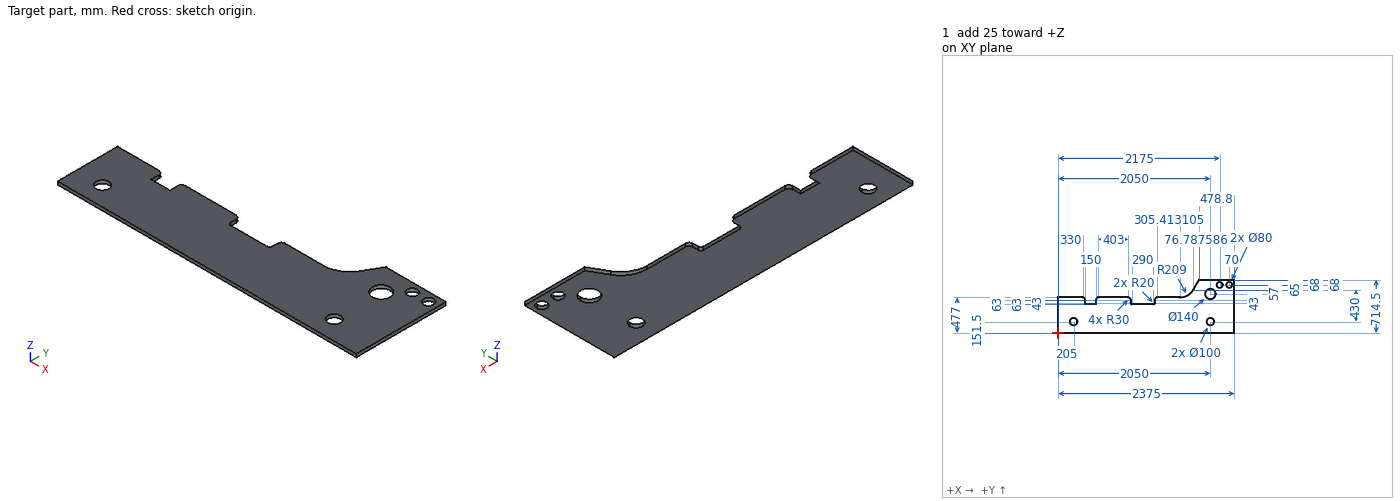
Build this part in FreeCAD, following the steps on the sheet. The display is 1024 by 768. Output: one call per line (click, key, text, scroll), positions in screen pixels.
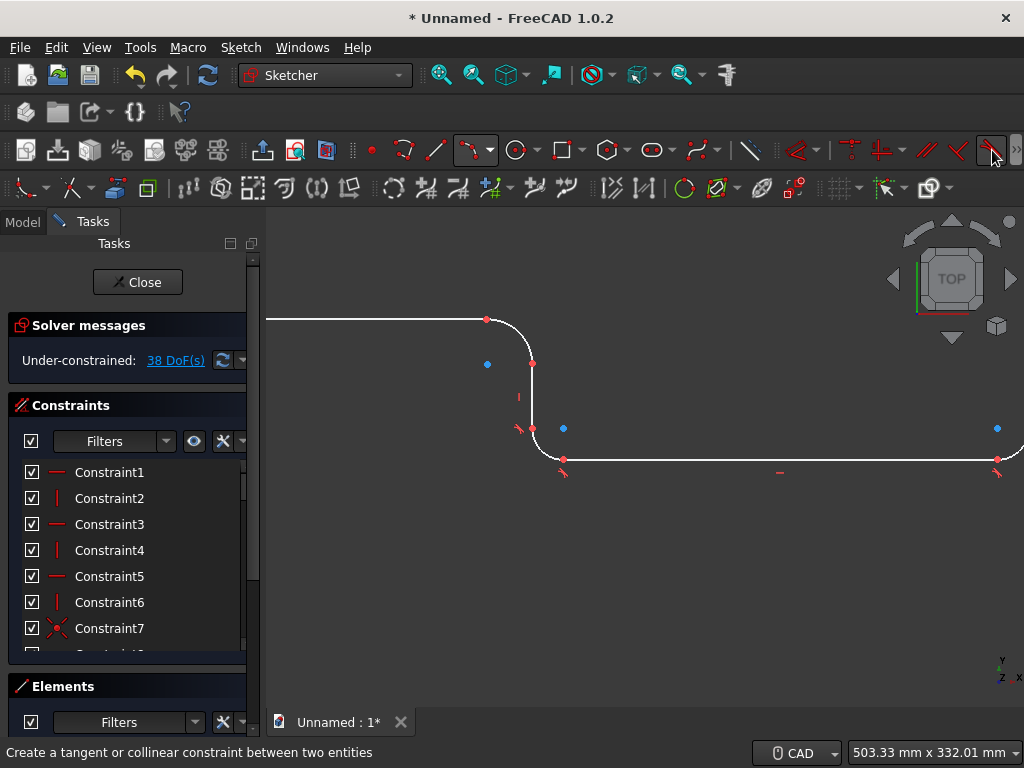
click(532, 409)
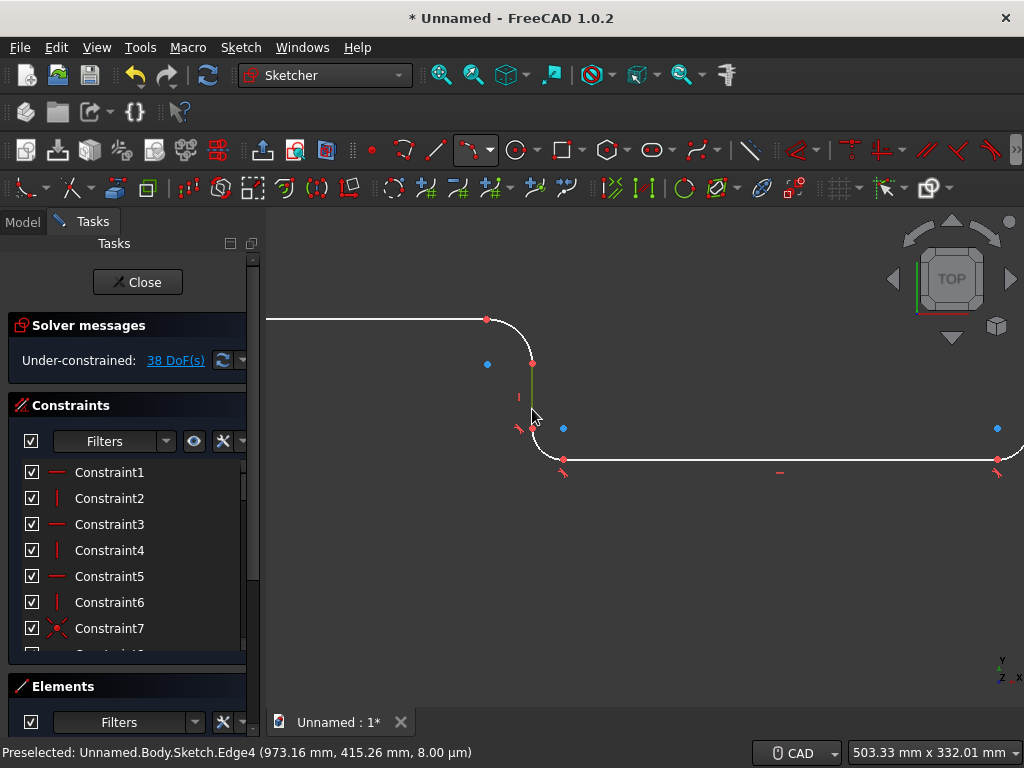
click(527, 343)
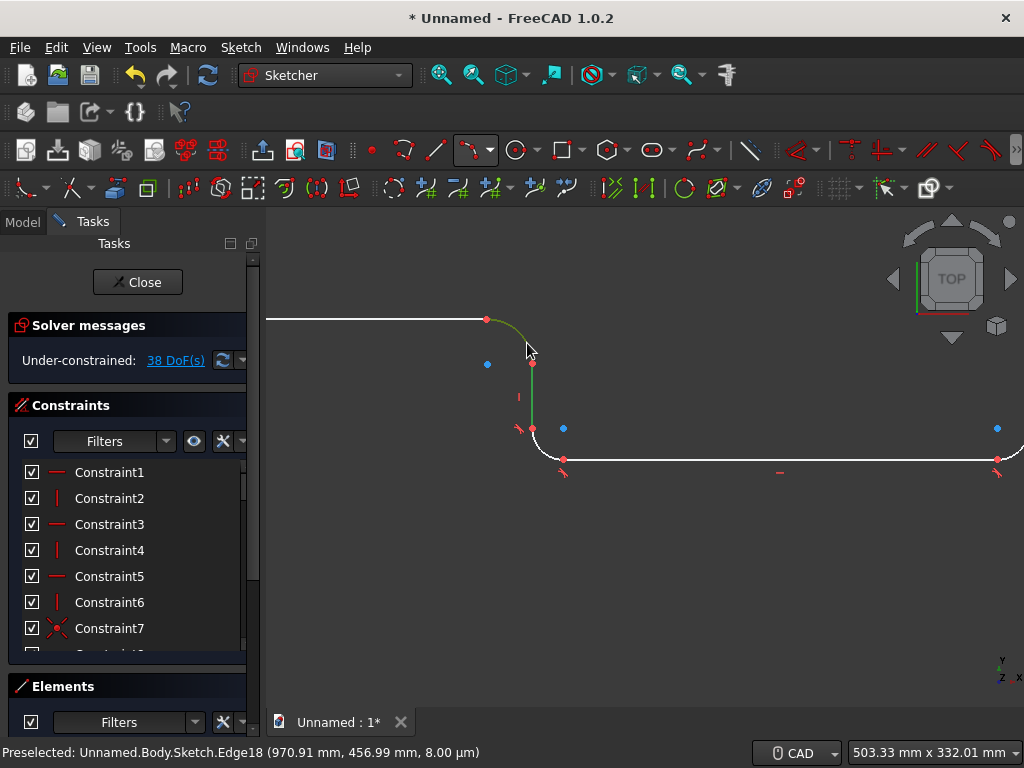
click(992, 150)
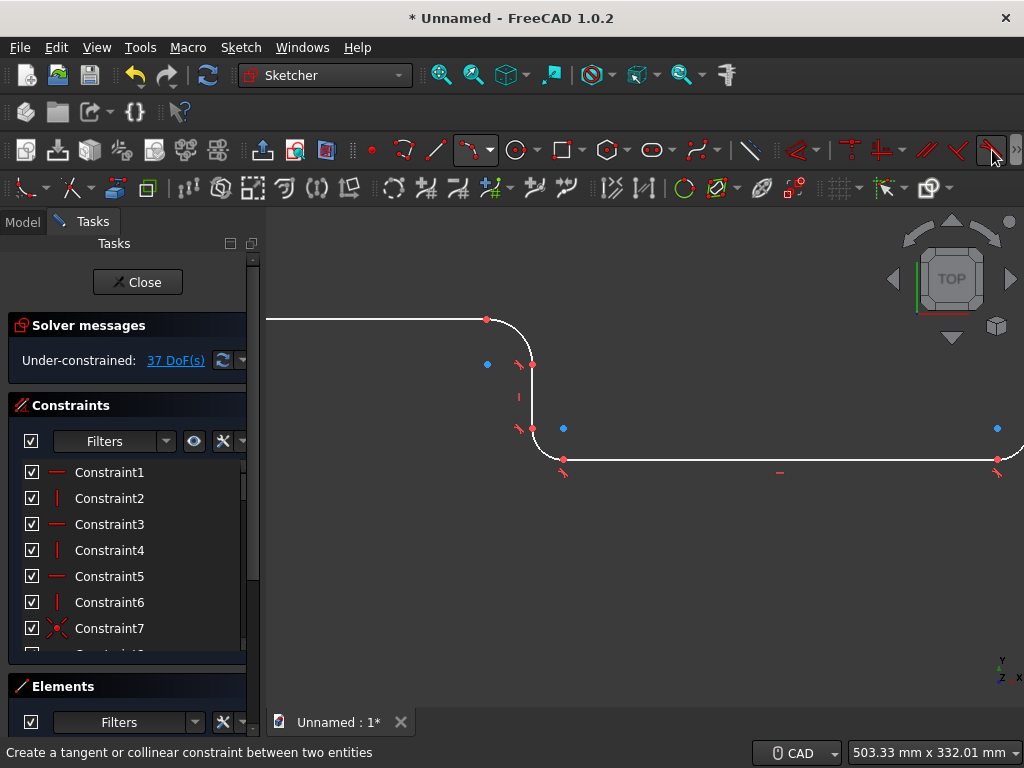
scroll(542, 452, down, 11)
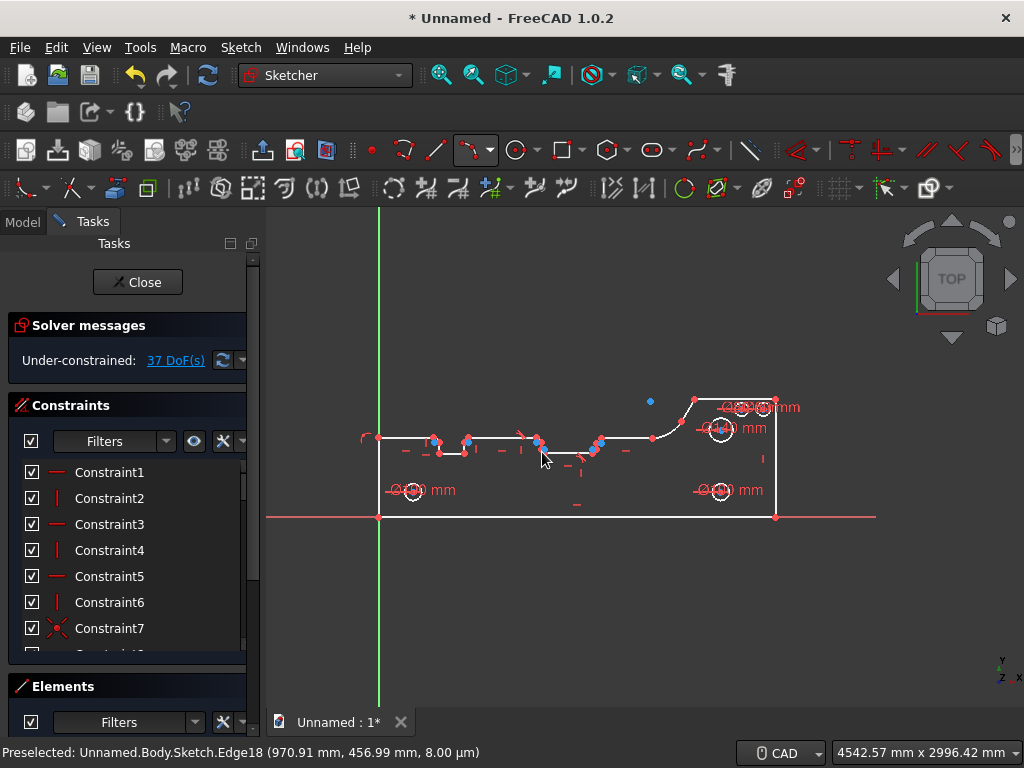
click(489, 438)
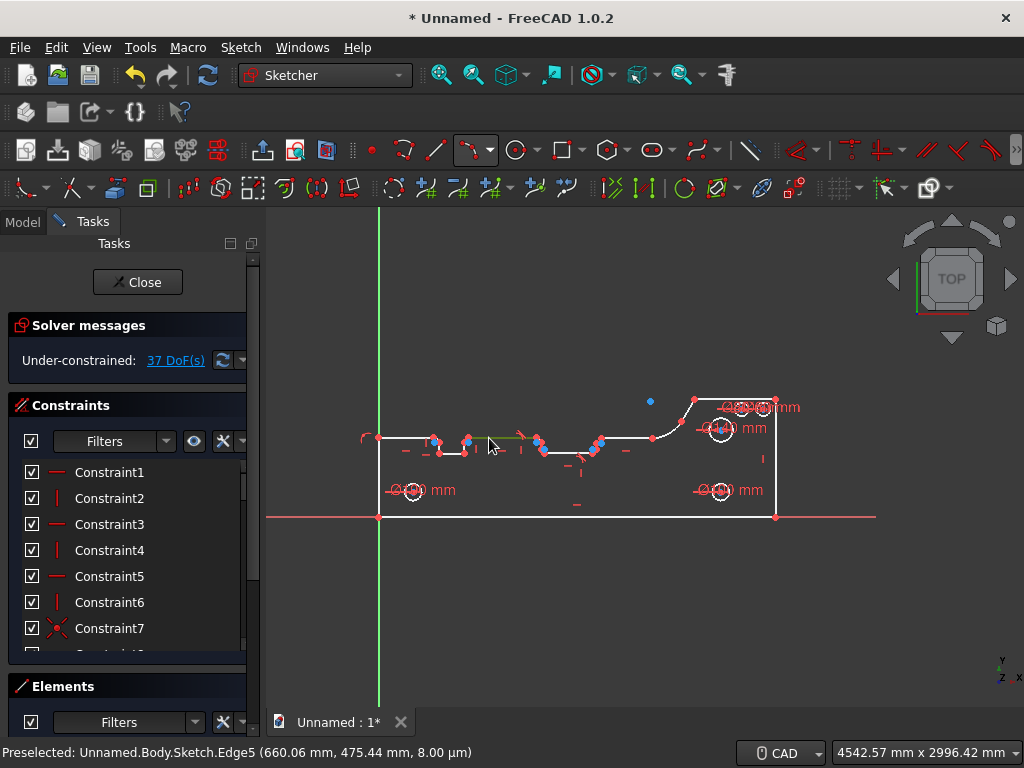
scroll(540, 439, up, 7)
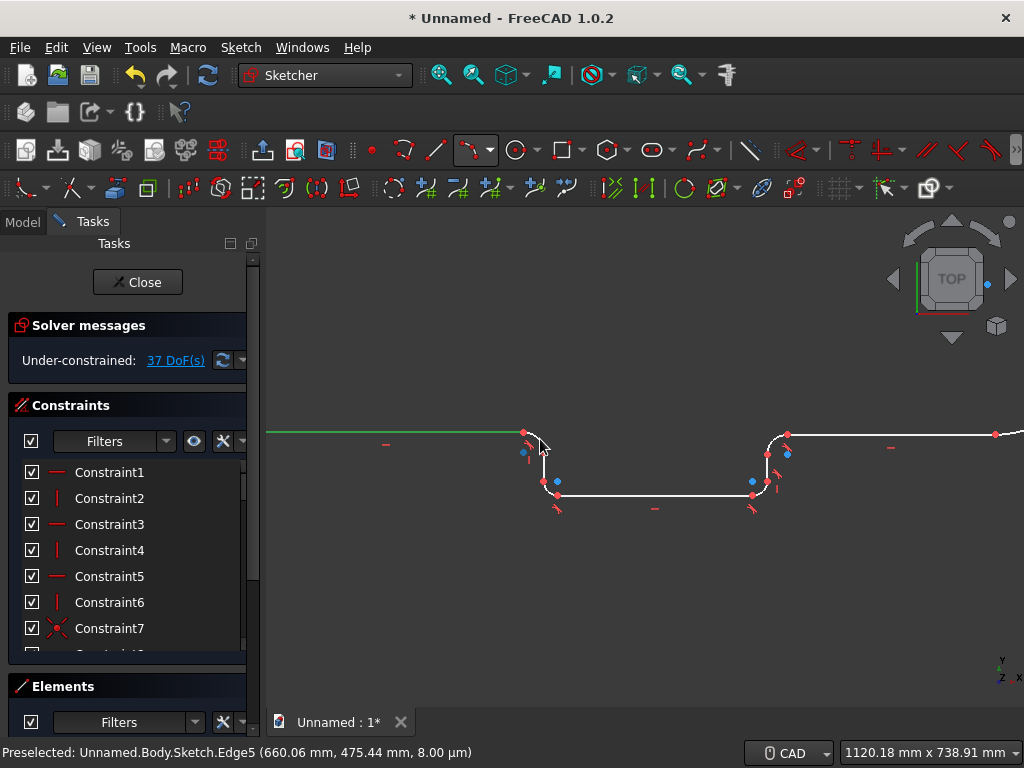
click(538, 438)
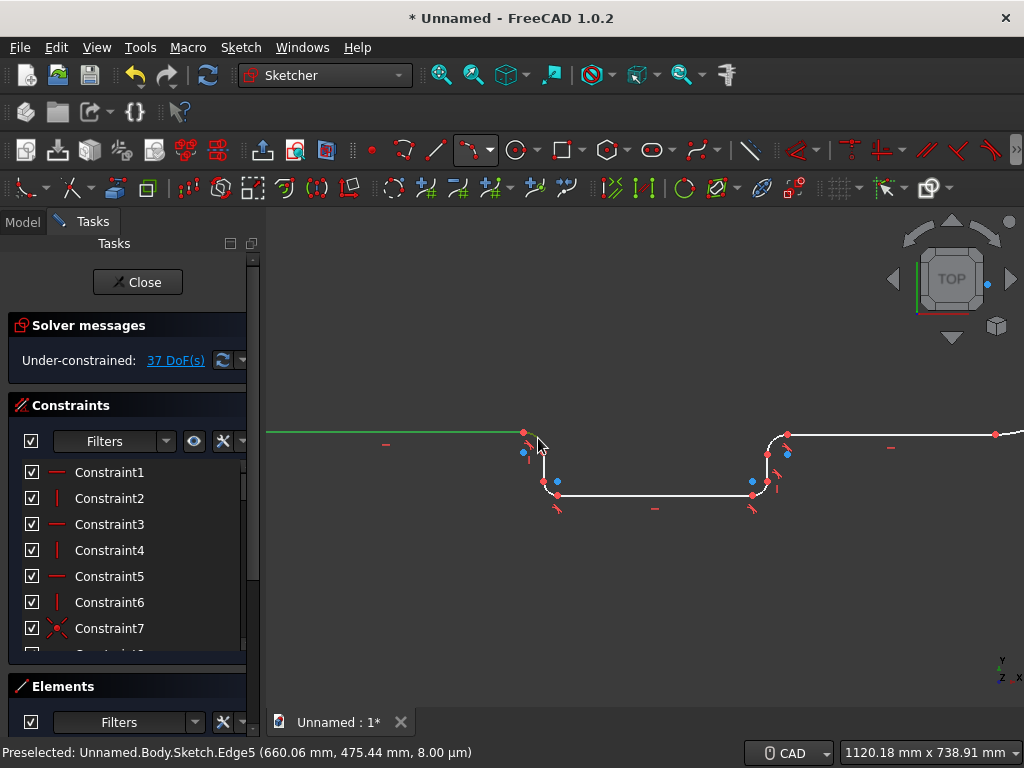
click(992, 150)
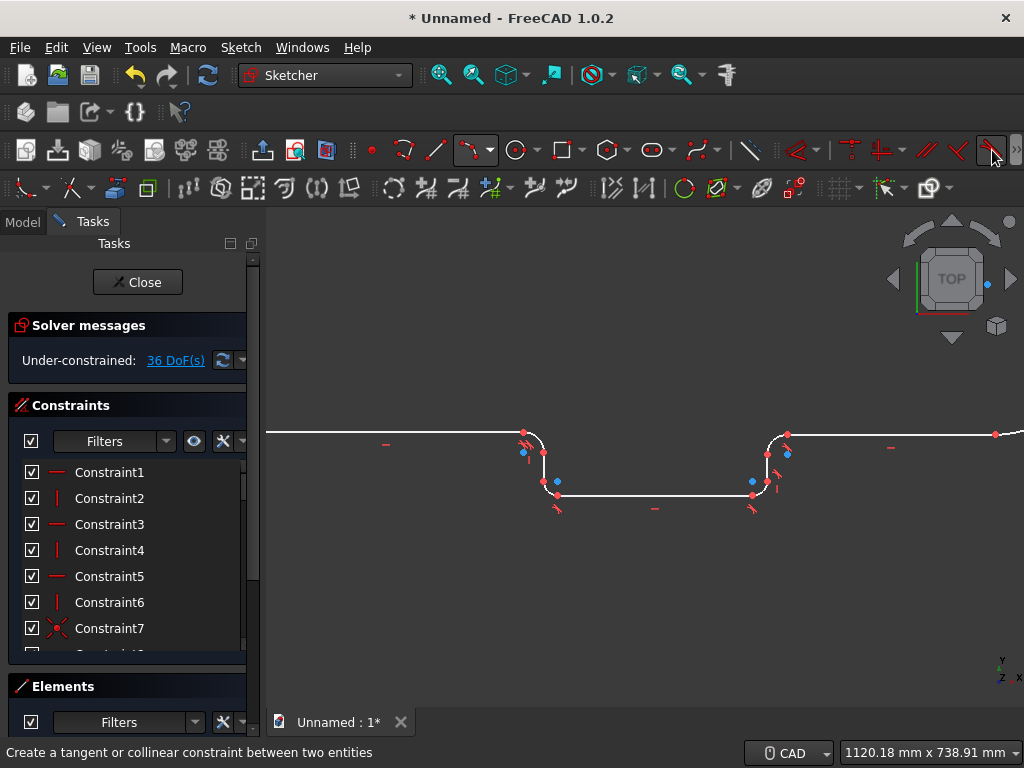
click(441, 432)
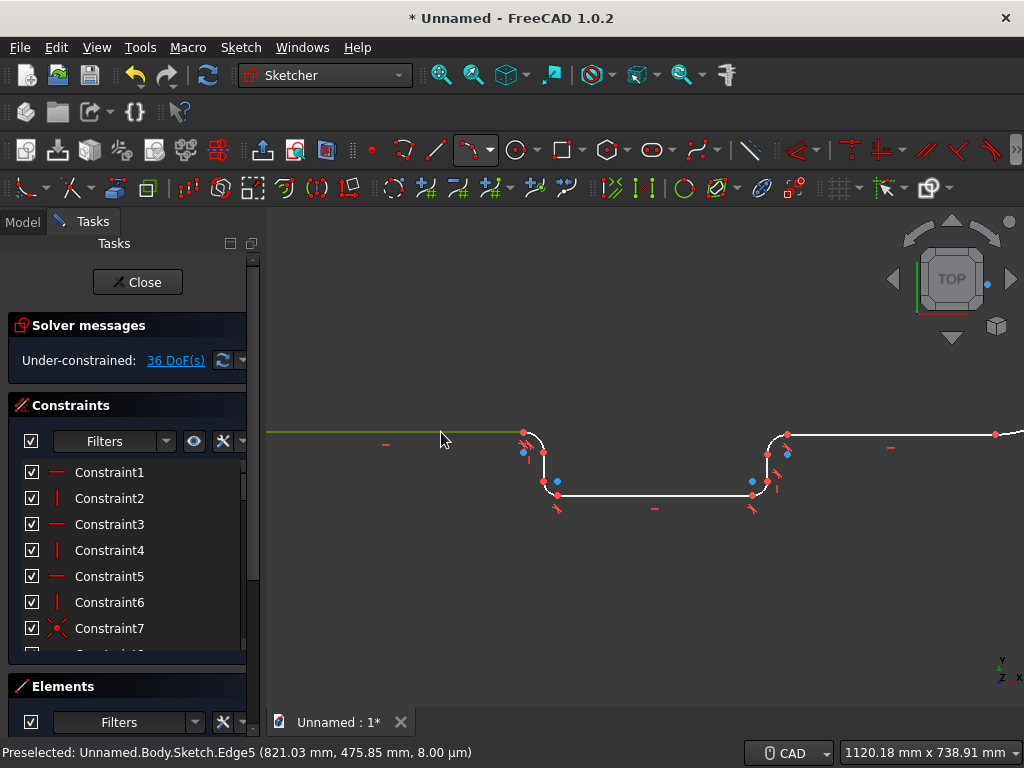
scroll(540, 439, down, 7)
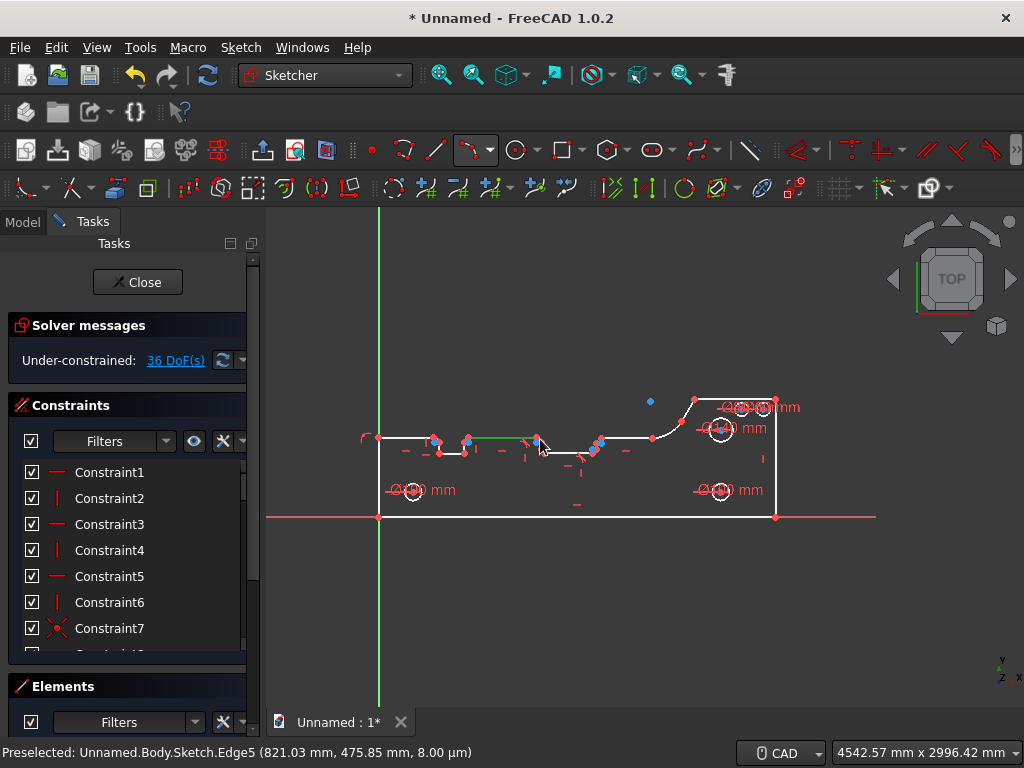
scroll(466, 438, up, 9)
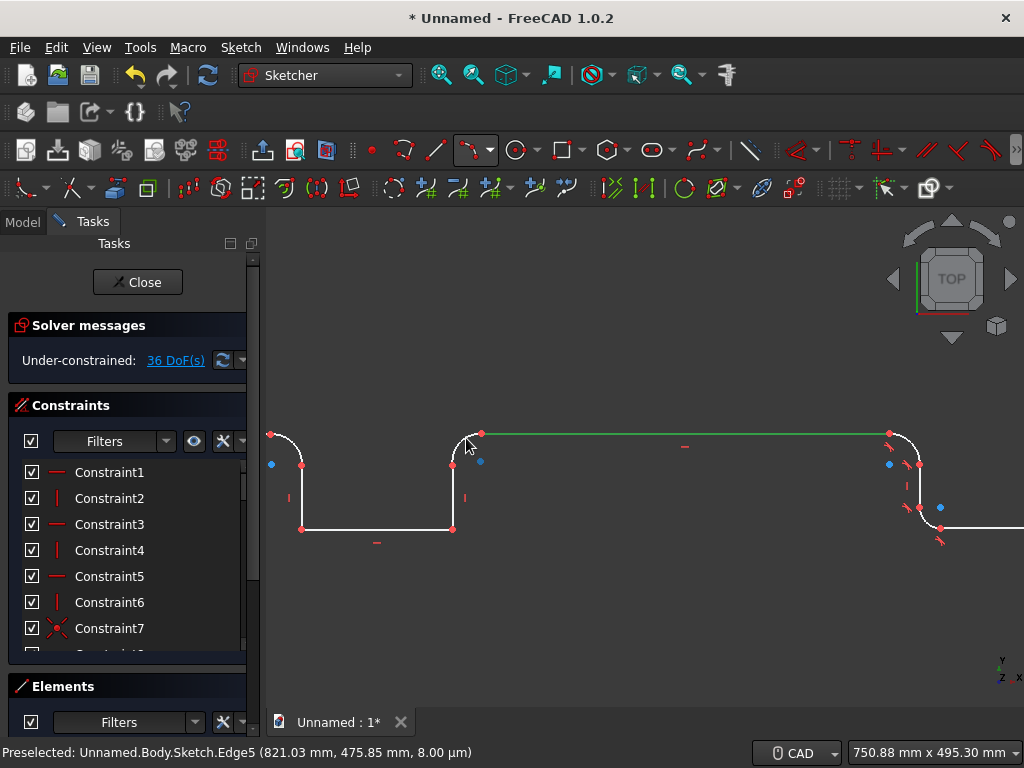
click(468, 437)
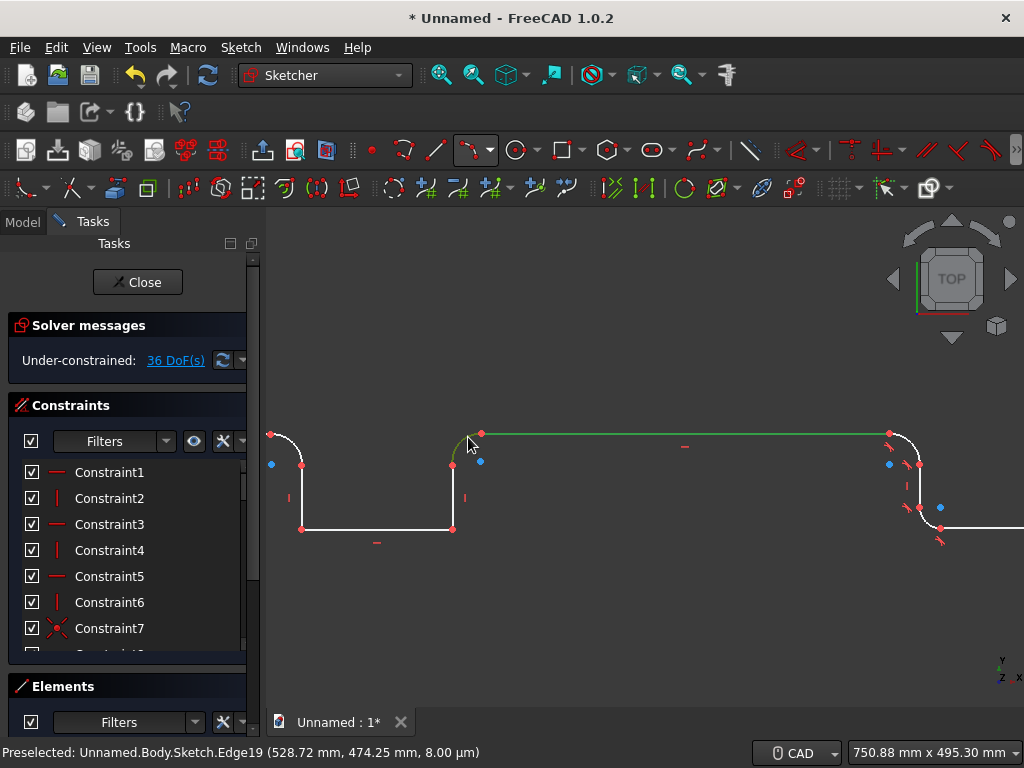
click(992, 150)